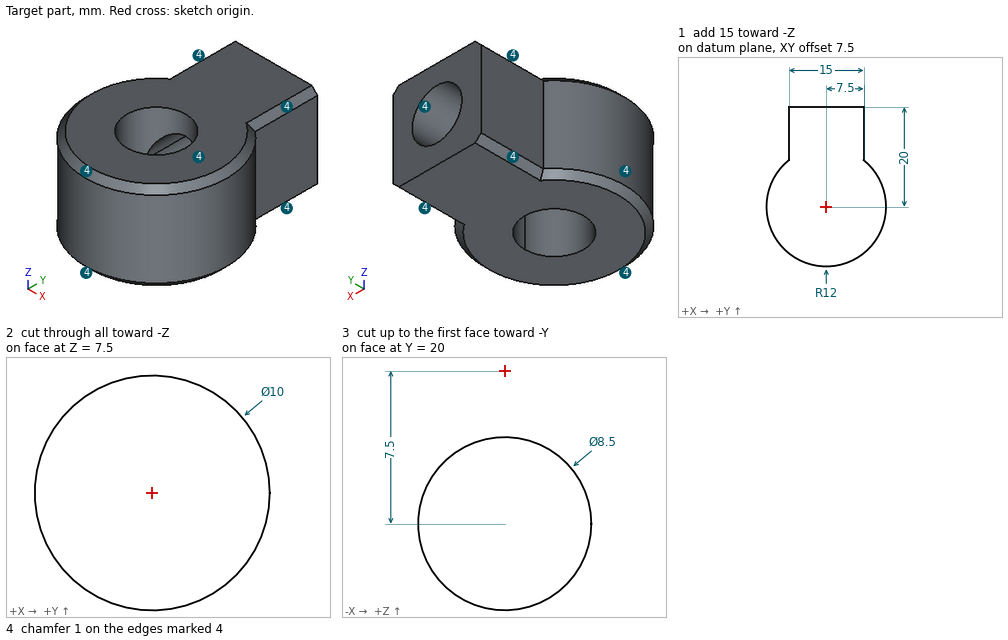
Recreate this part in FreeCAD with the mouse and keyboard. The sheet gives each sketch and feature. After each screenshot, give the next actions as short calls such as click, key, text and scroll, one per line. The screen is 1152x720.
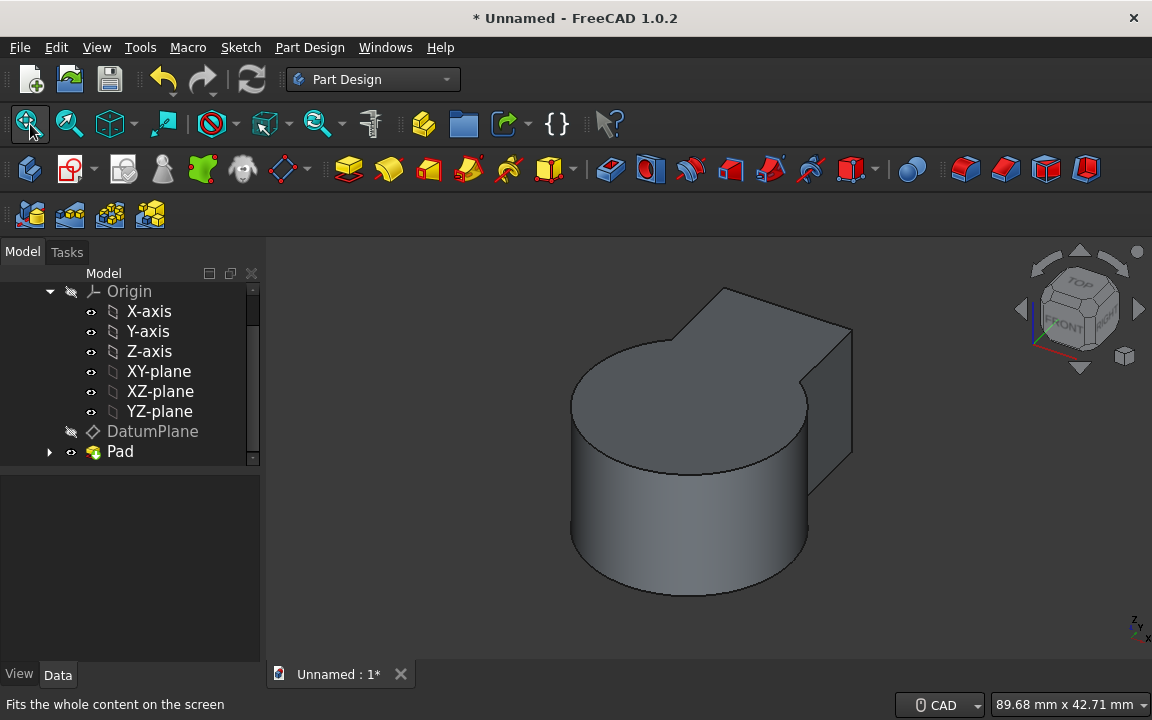
click(686, 409)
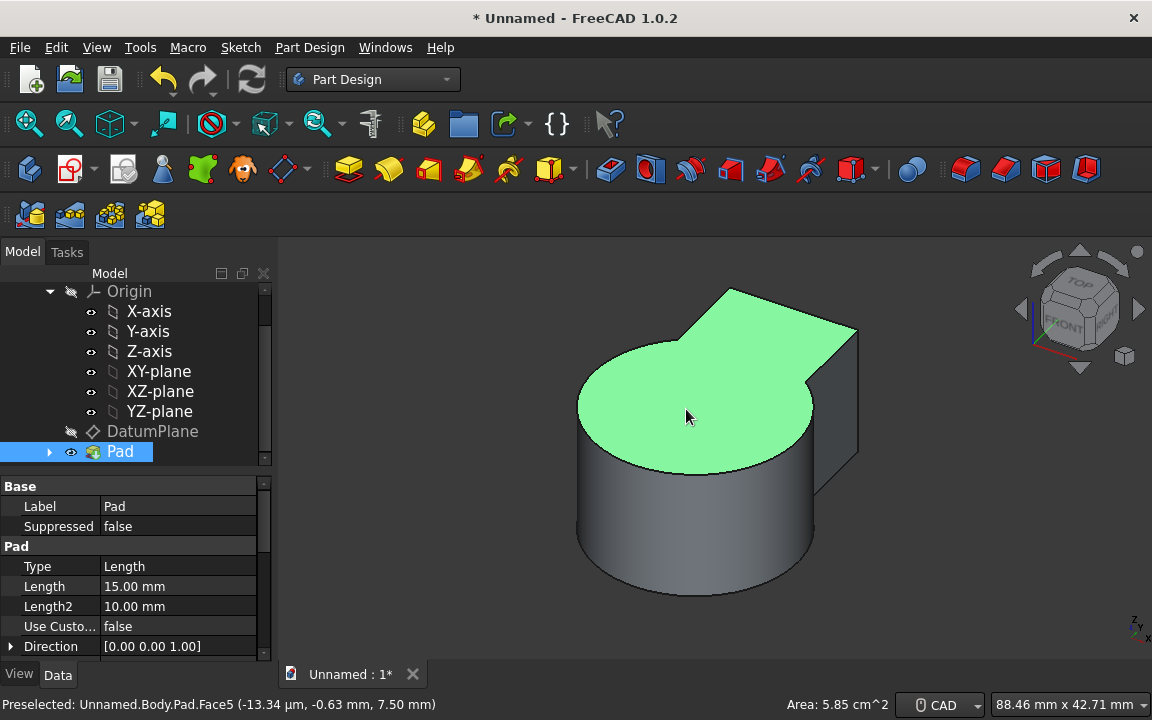
click(70, 170)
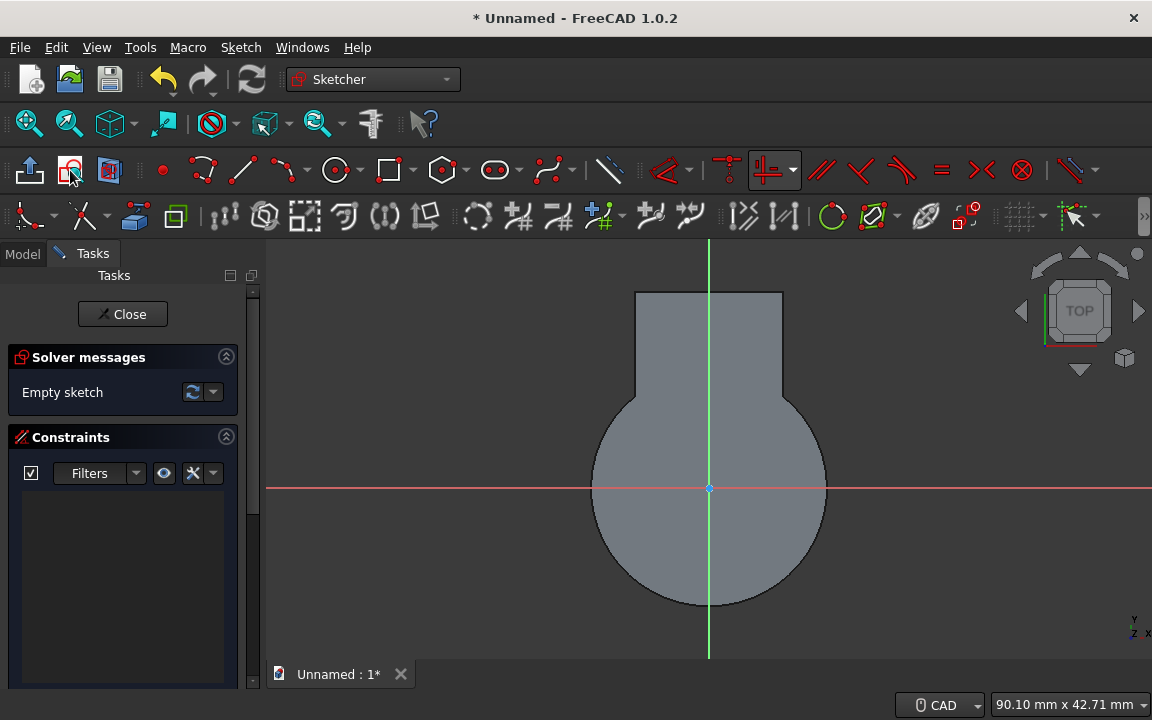
scroll(749, 511, up, 5)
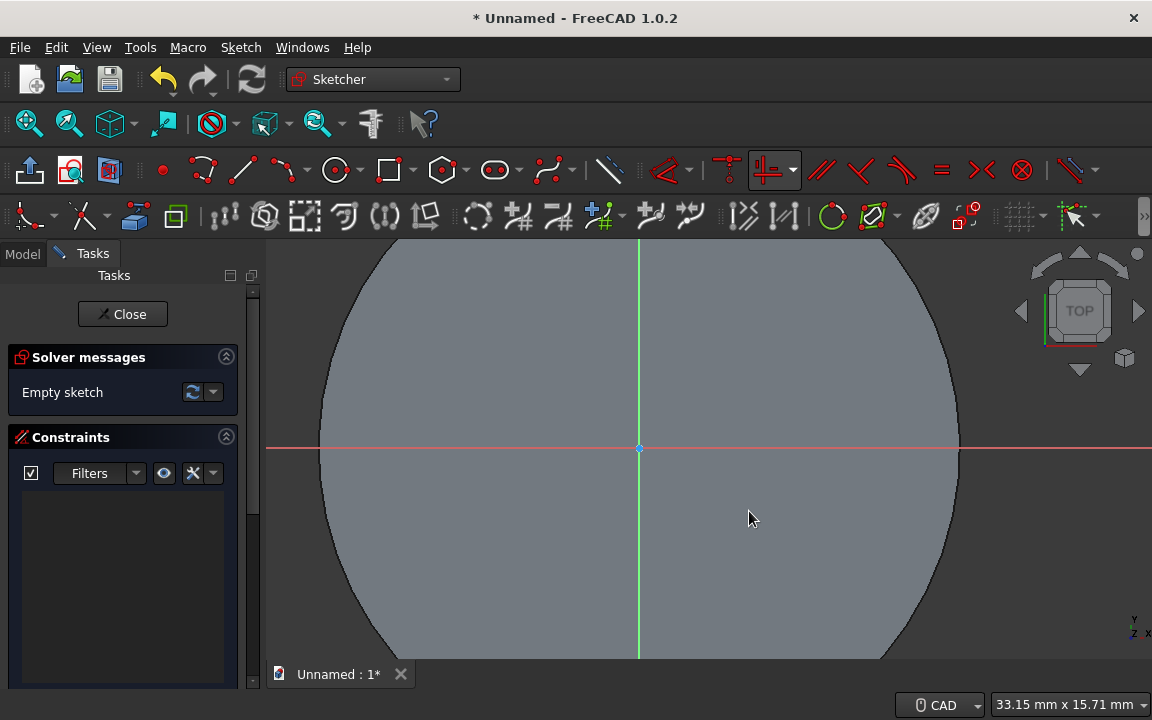
click(336, 170)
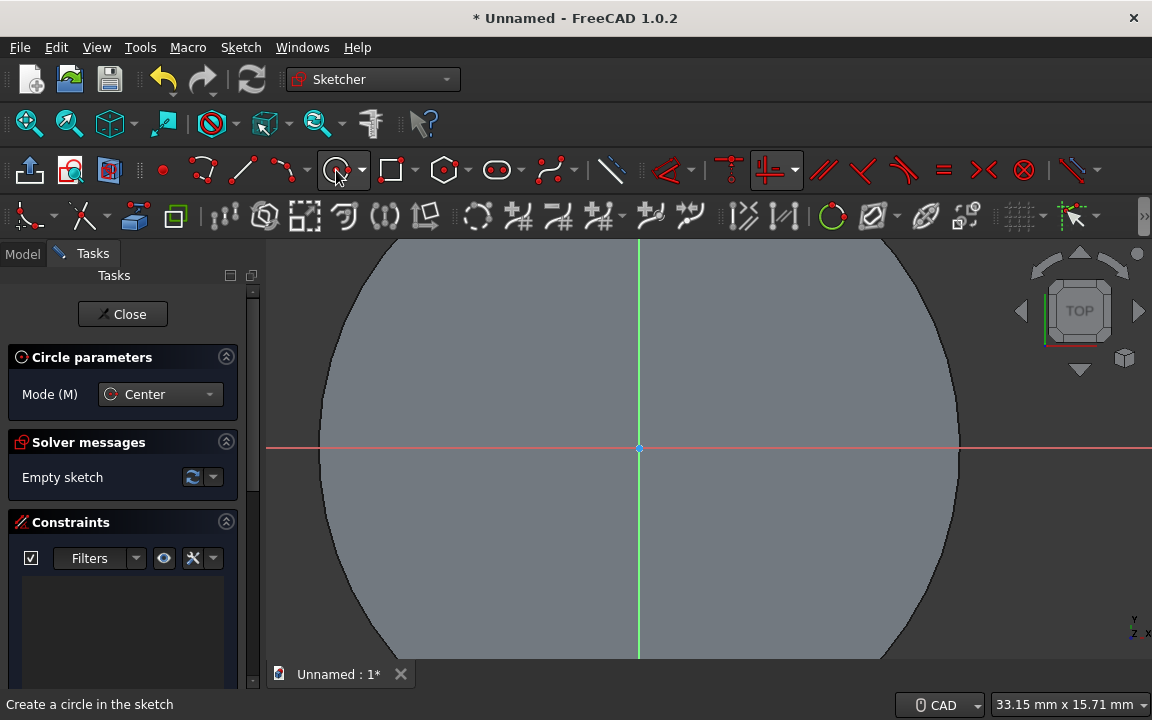
click(639, 448)
click(734, 354)
key(Escape)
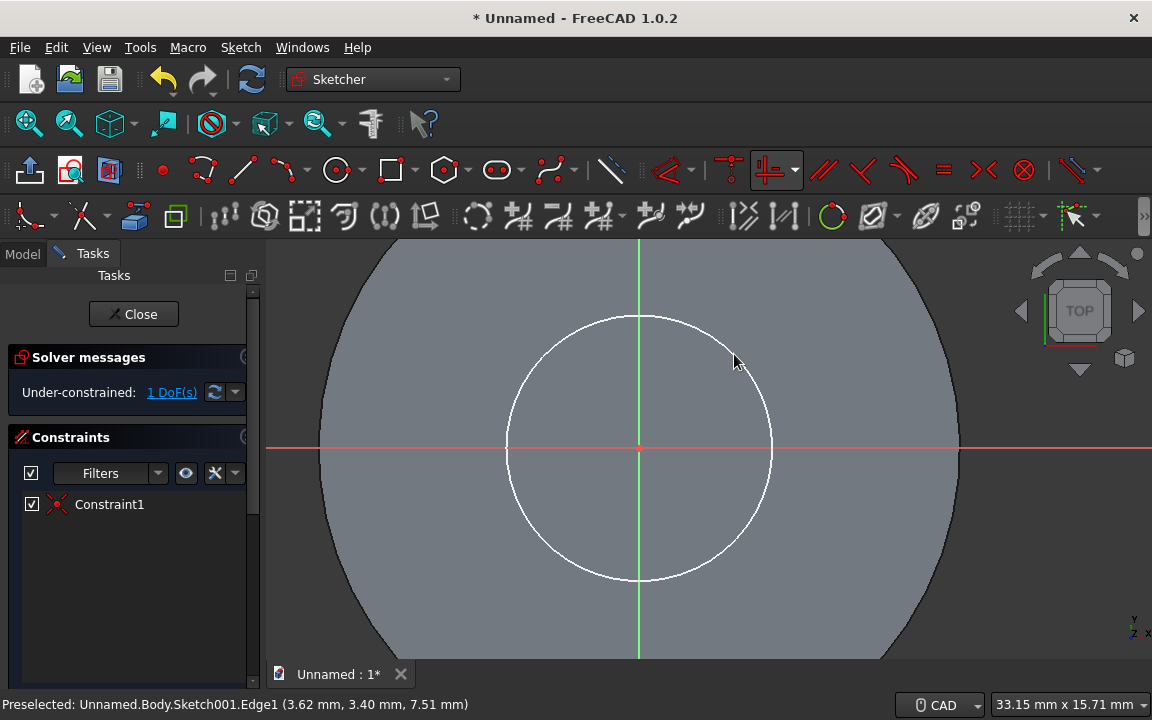
click(666, 170)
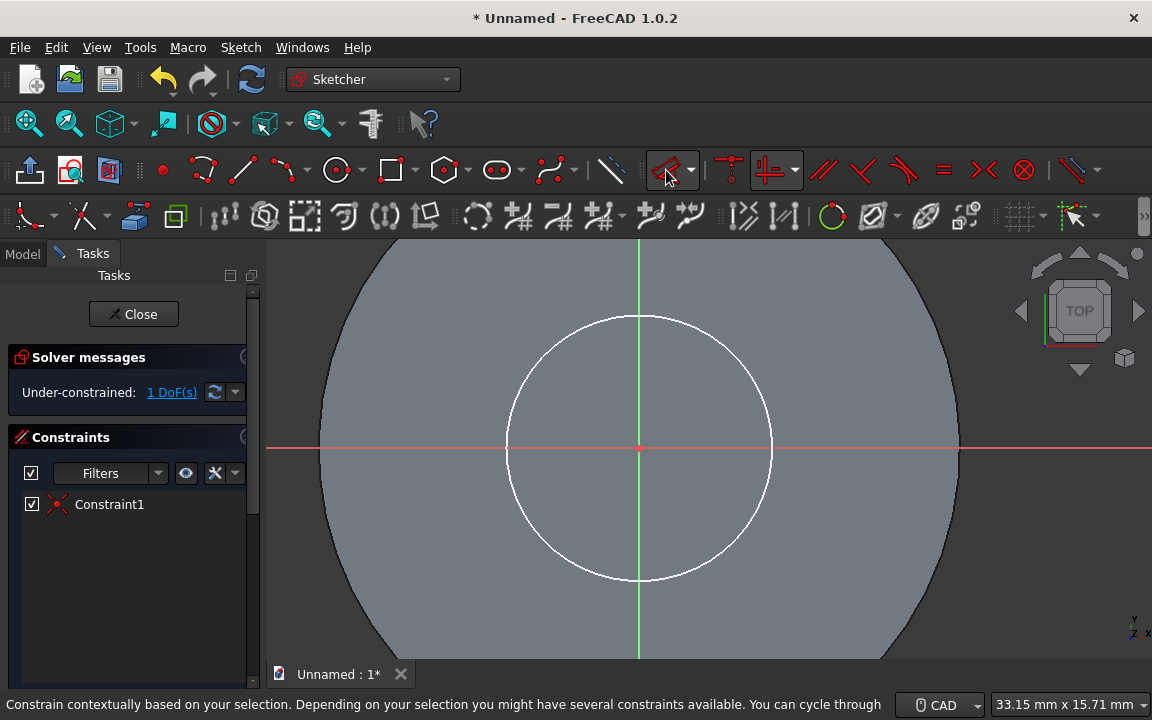
click(733, 354)
click(756, 331)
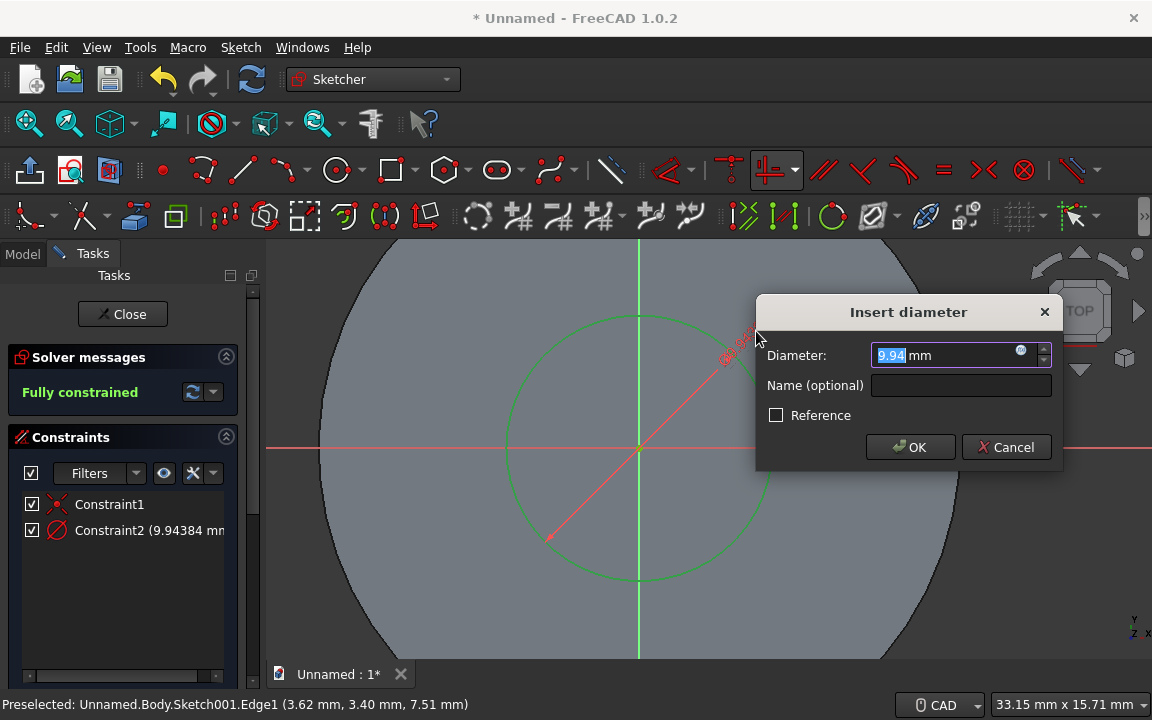
text(10)
key(Return)
key(Escape)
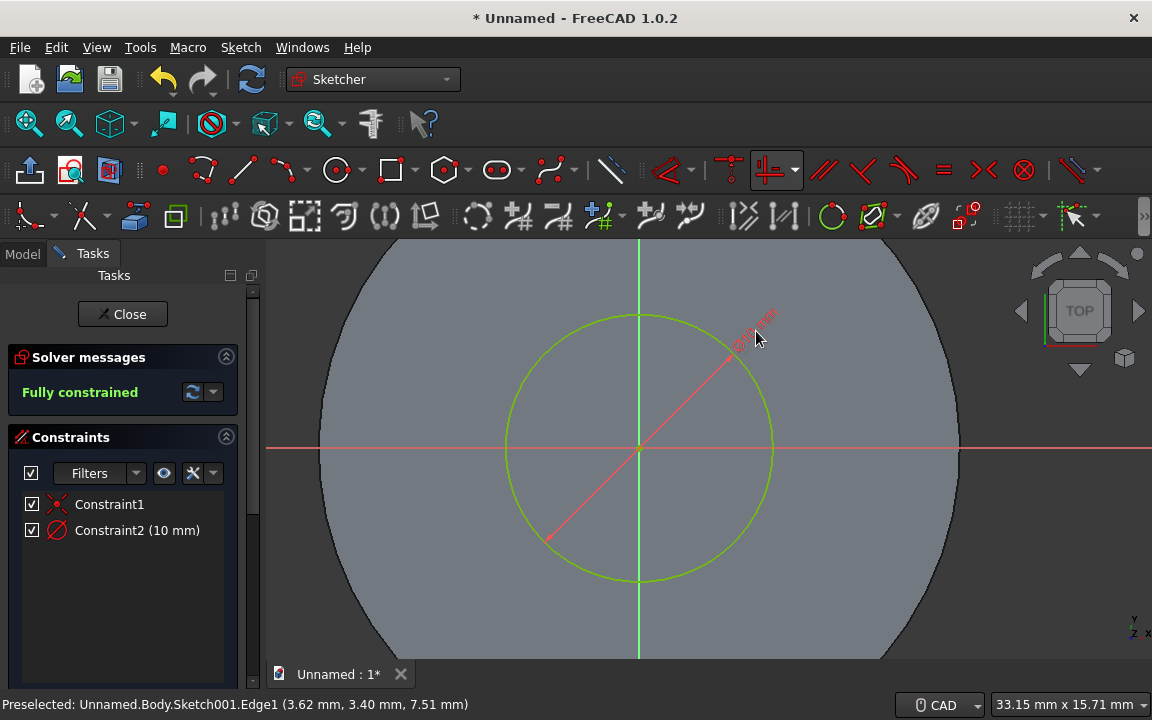
click(123, 314)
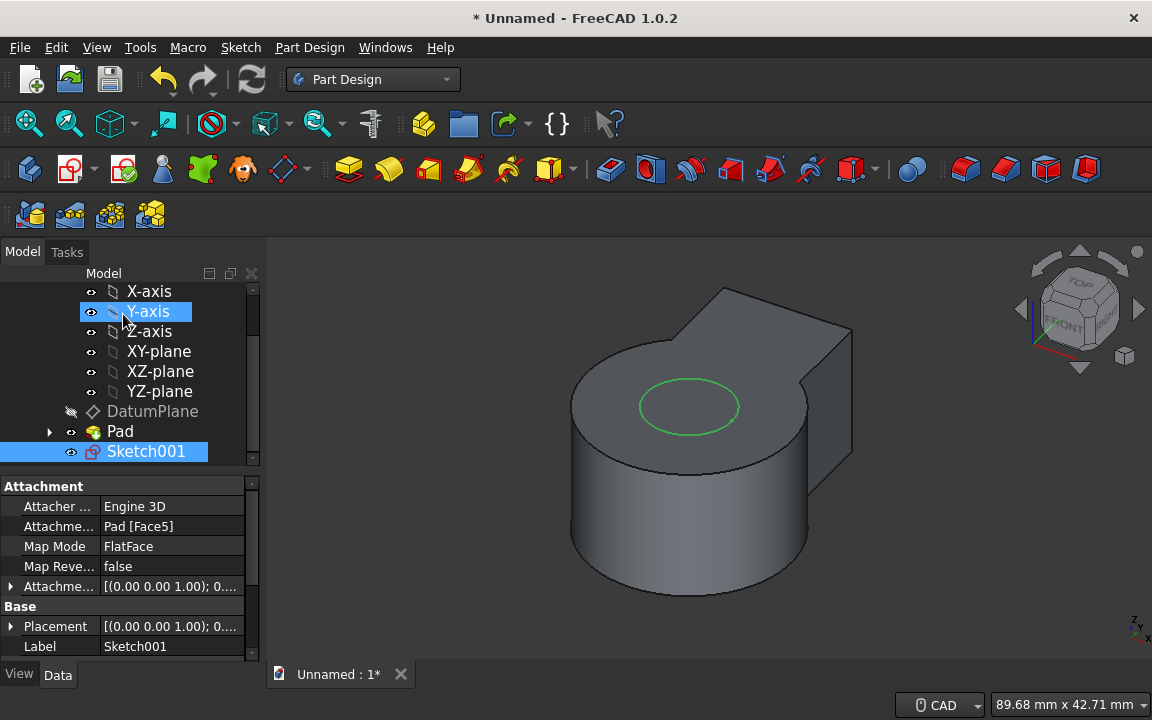
click(612, 170)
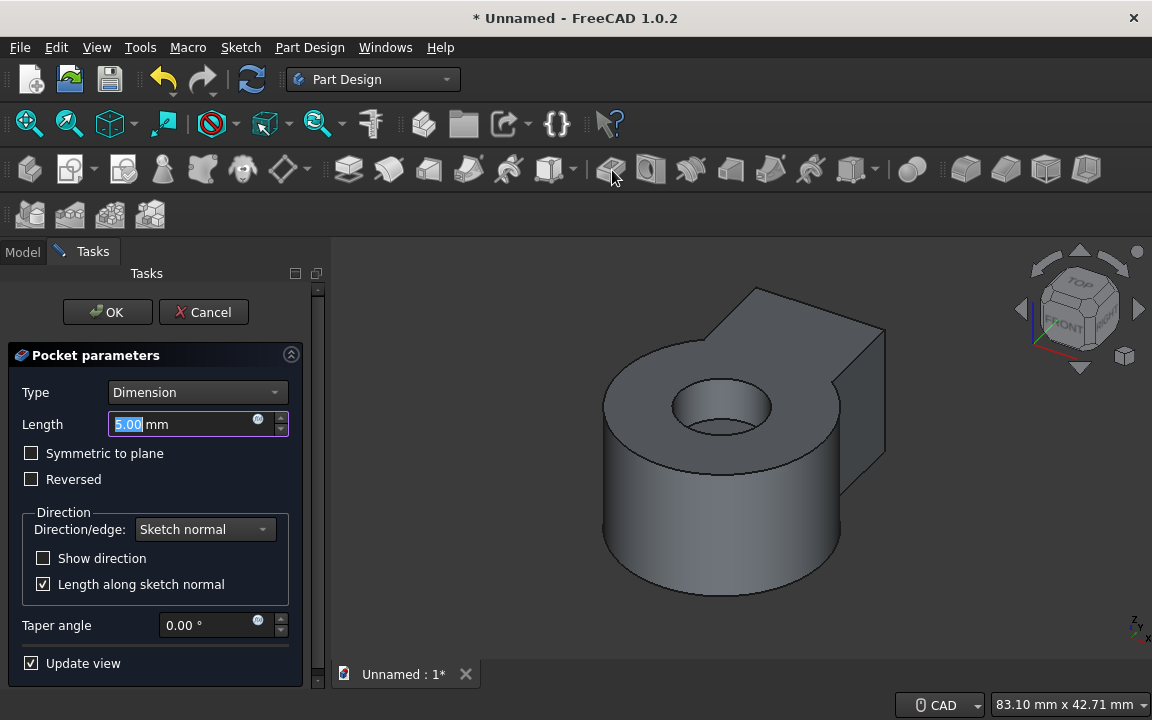
click(198, 392)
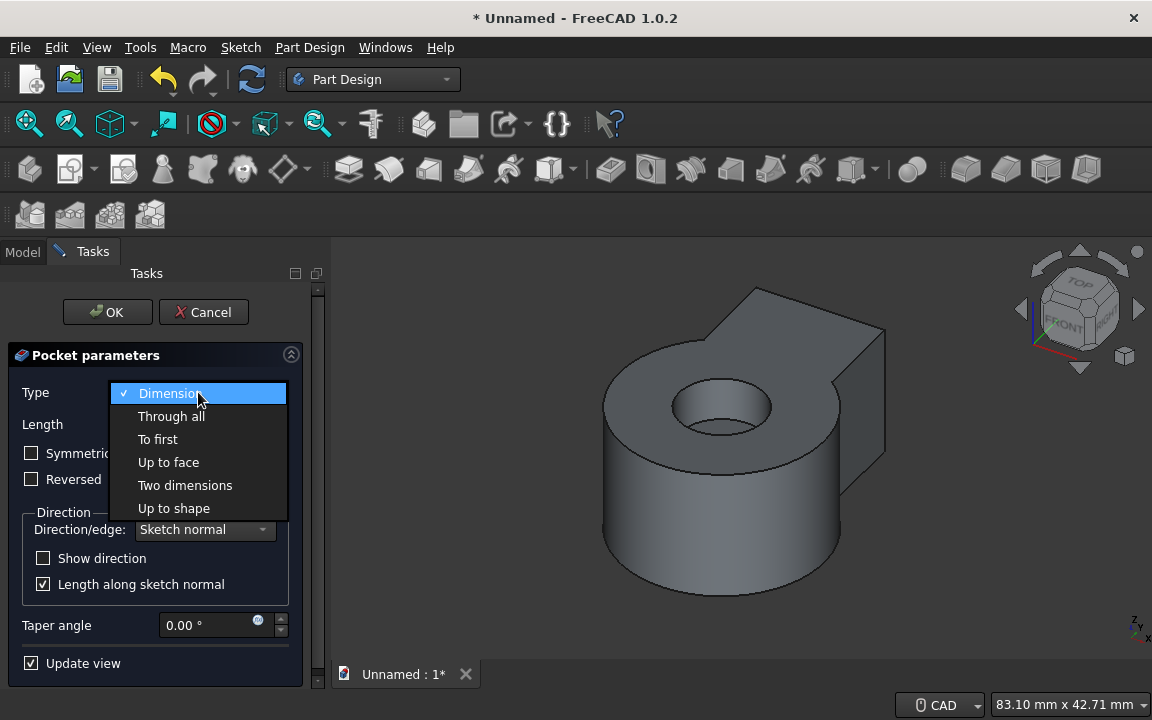
click(198, 416)